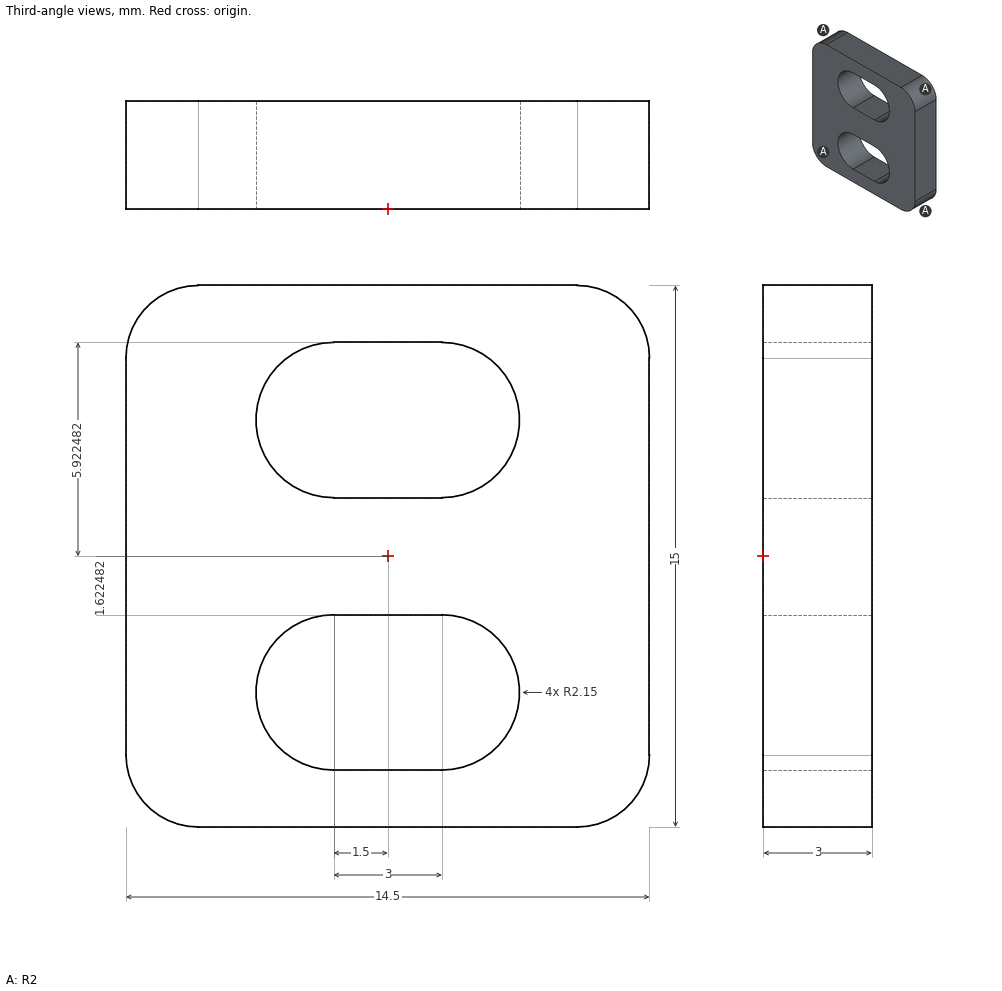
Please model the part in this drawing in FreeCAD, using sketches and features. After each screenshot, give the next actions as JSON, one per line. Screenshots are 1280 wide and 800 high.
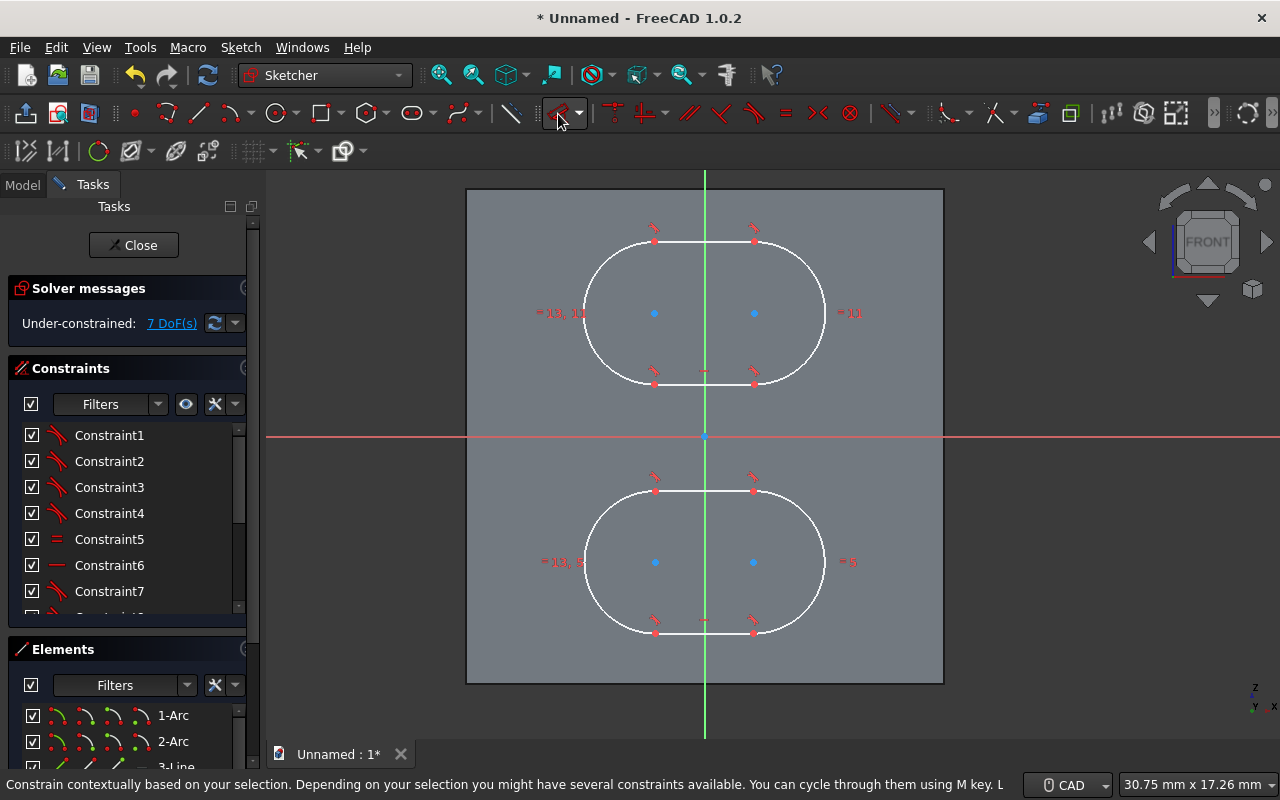
{"action": "left_click", "coordinate": [598, 520]}
{"action": "left_click", "coordinate": [572, 501]}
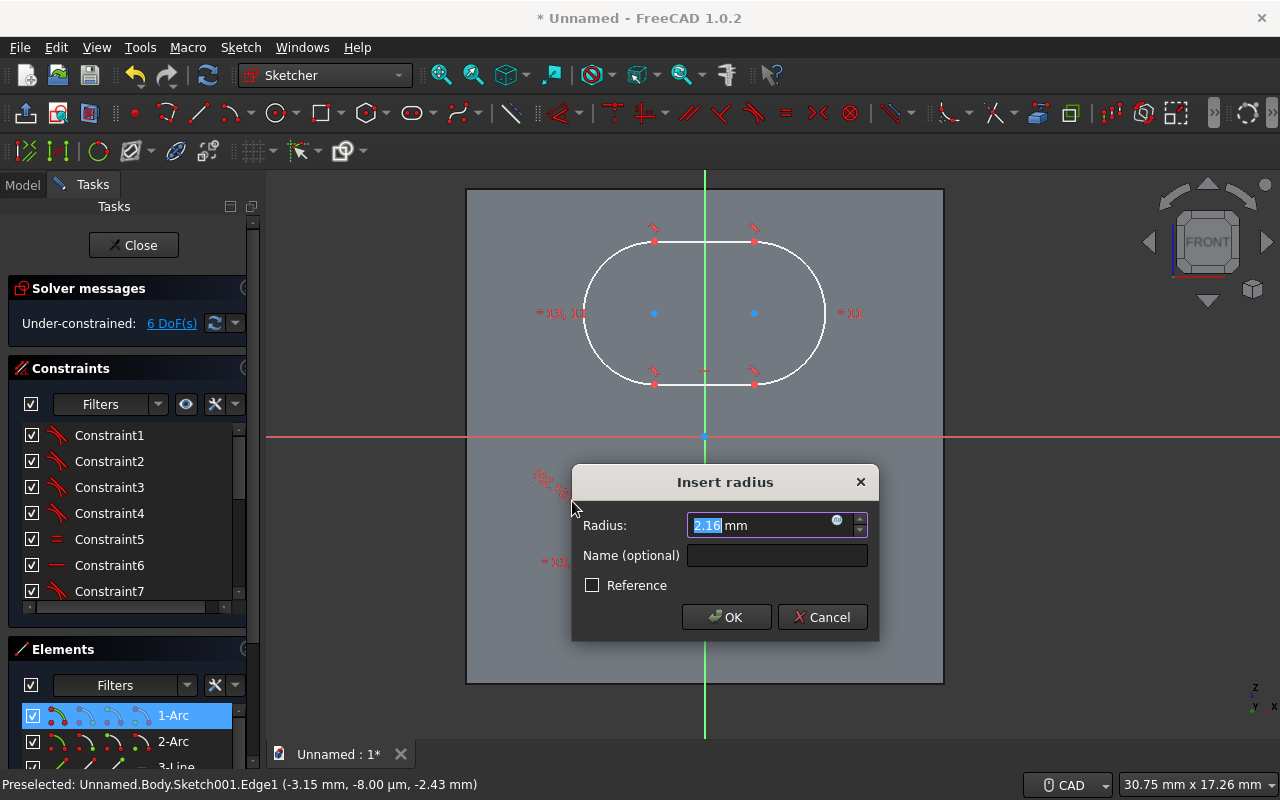
{"action": "type", "text": "2.15"}
{"action": "key", "text": "Return"}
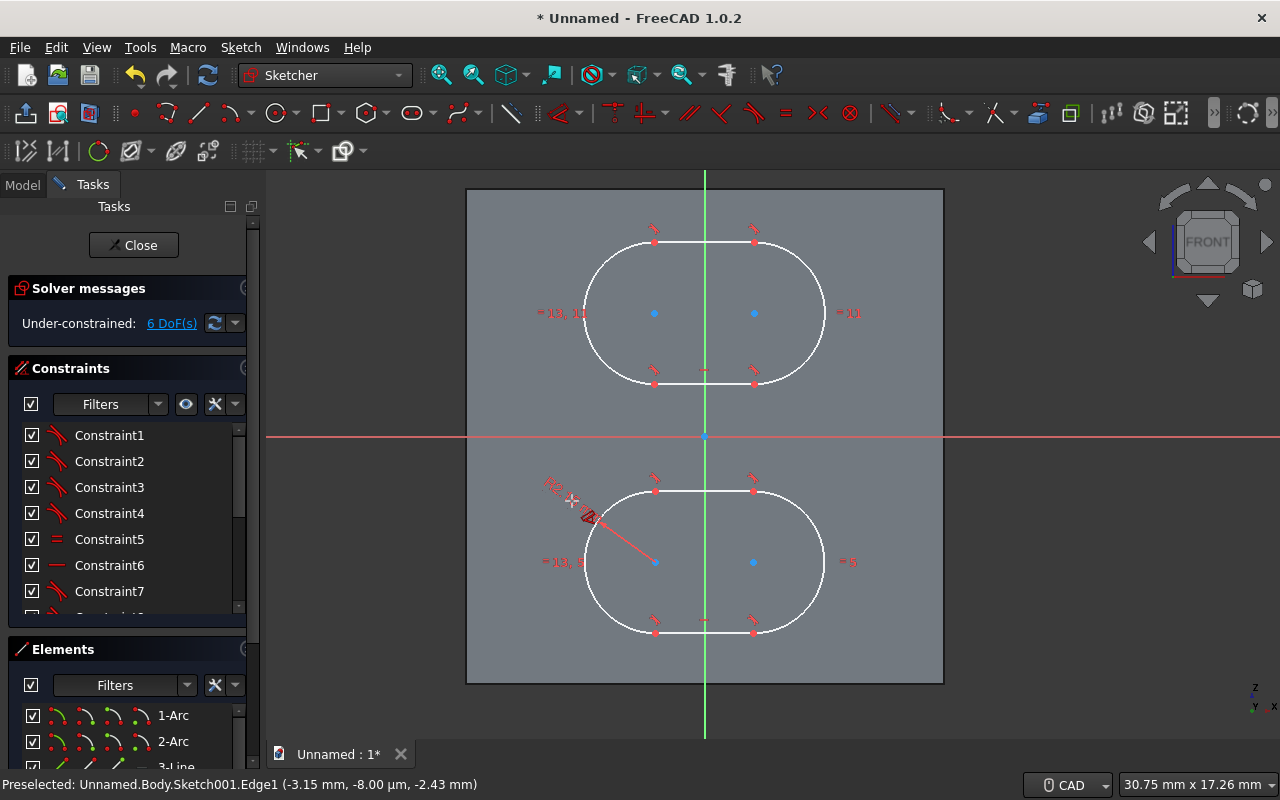
{"action": "left_click", "coordinate": [685, 491]}
{"action": "left_click", "coordinate": [682, 525]}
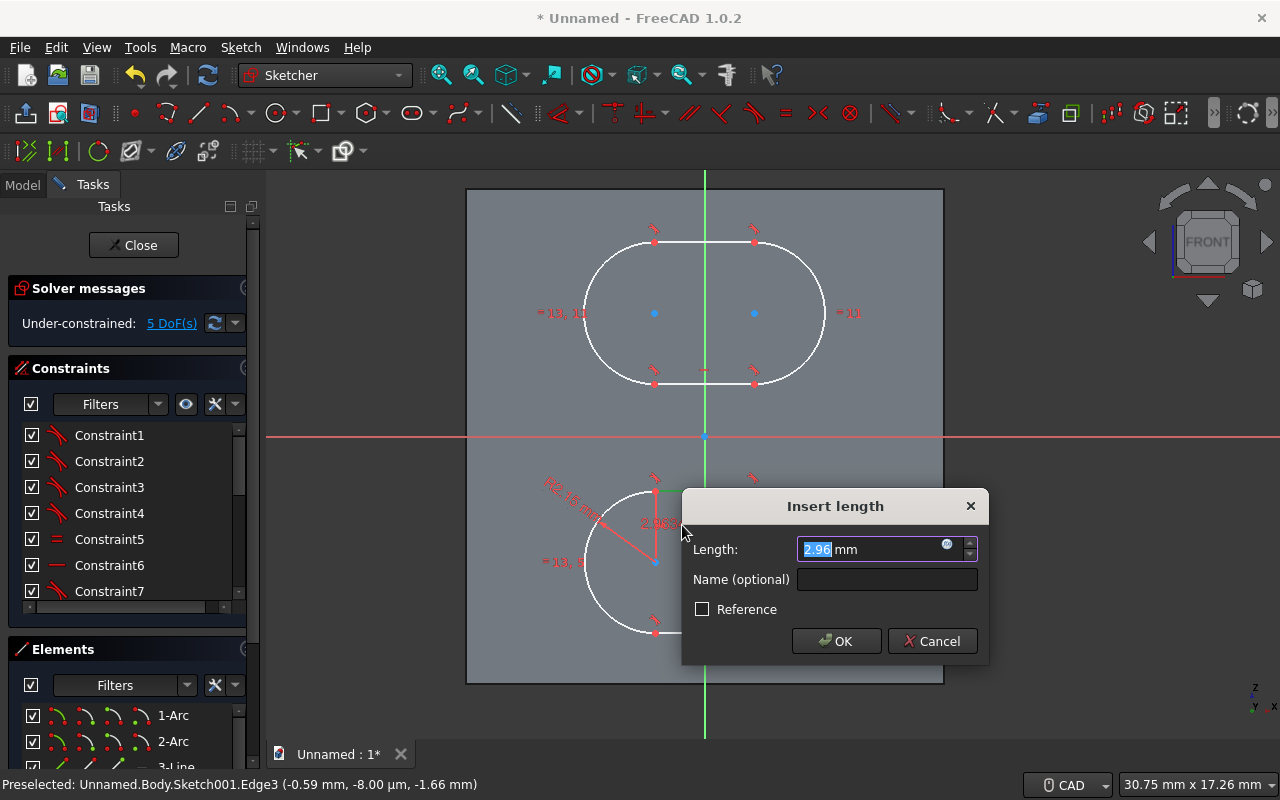
{"action": "type", "text": "3"}
{"action": "key", "text": "Return"}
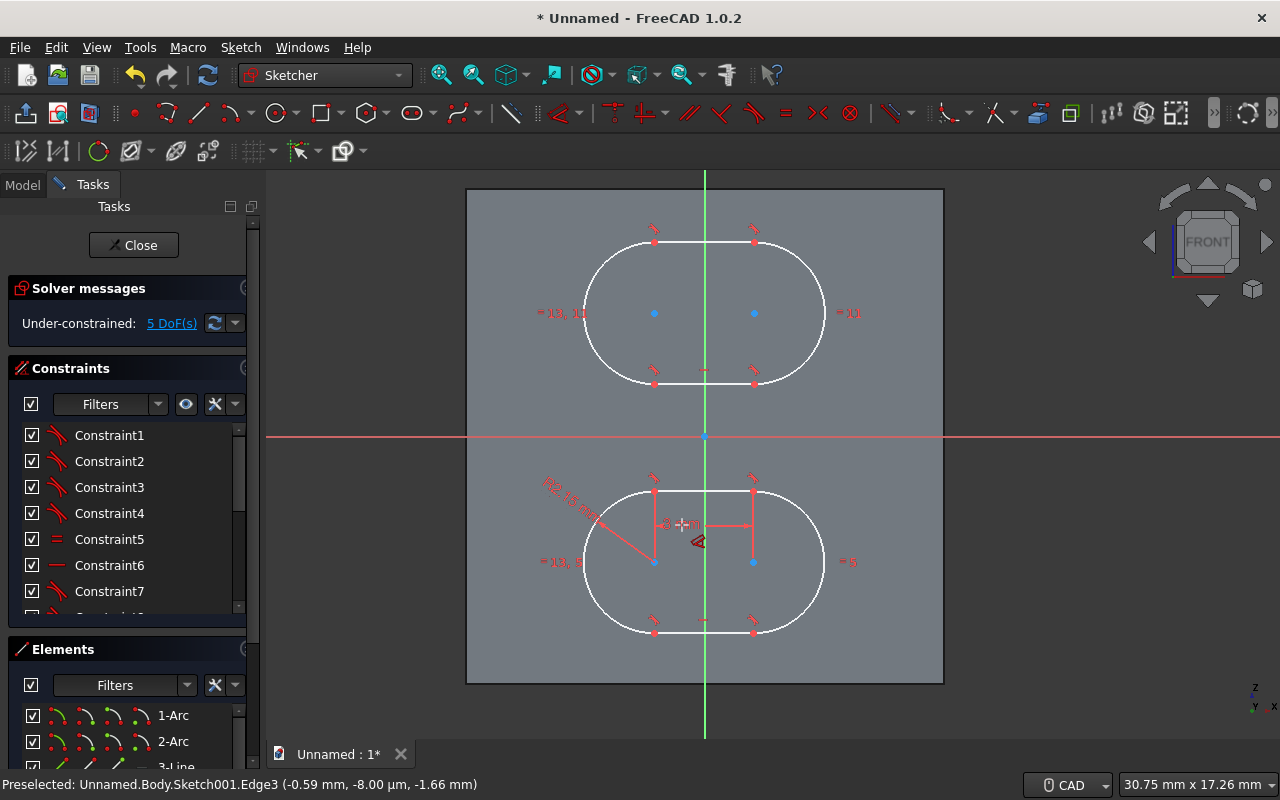
{"action": "left_click", "coordinate": [685, 242]}
{"action": "left_click", "coordinate": [682, 208]}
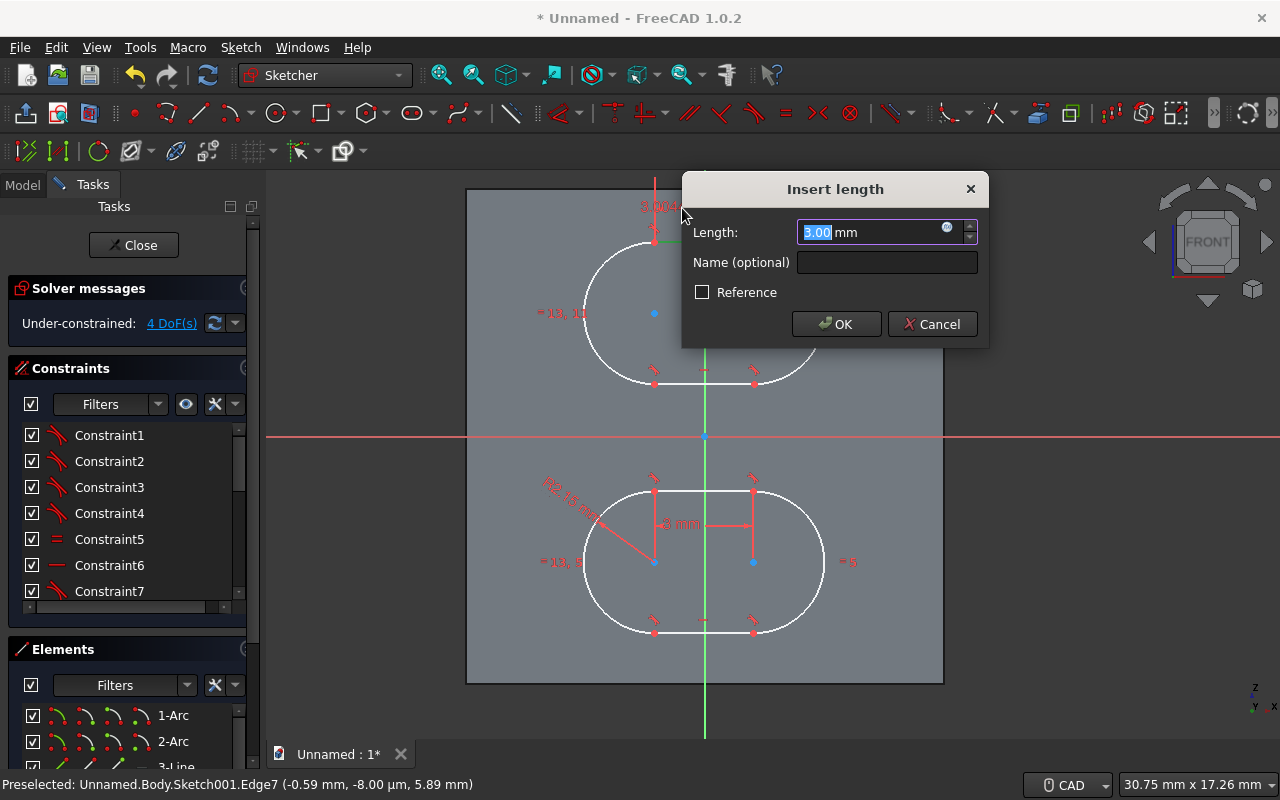
{"action": "type", "text": "3"}
{"action": "key", "text": "Return"}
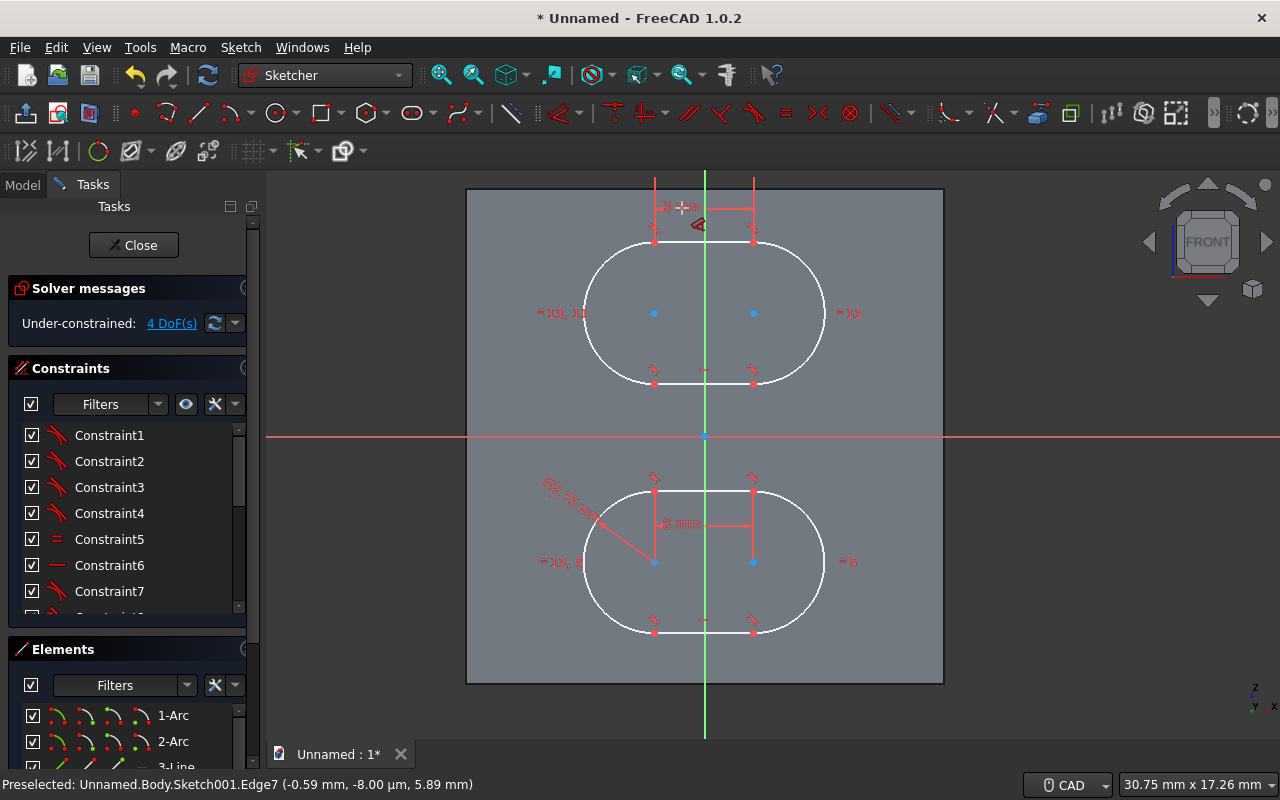
{"action": "left_click", "coordinate": [655, 491]}
{"action": "left_click", "coordinate": [680, 403]}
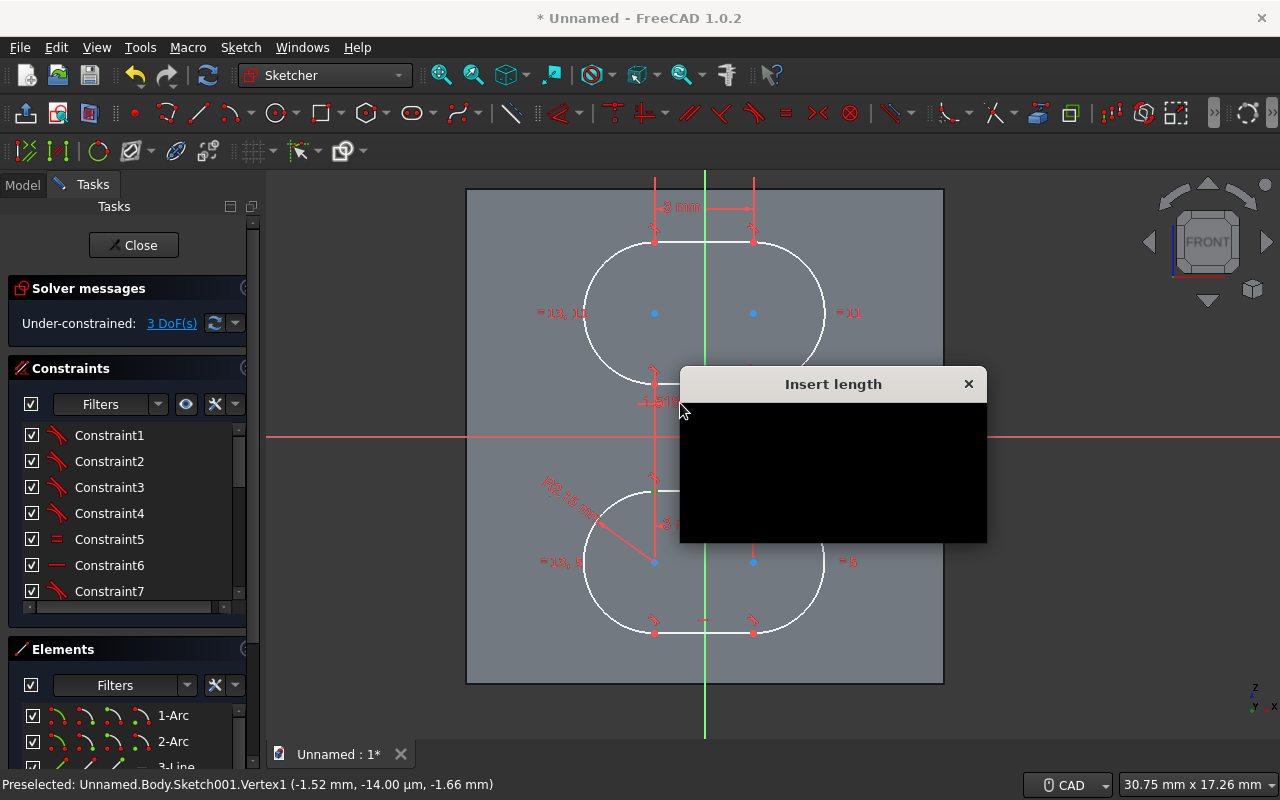
{"action": "type", "text": "1.5"}
{"action": "key", "text": "Return"}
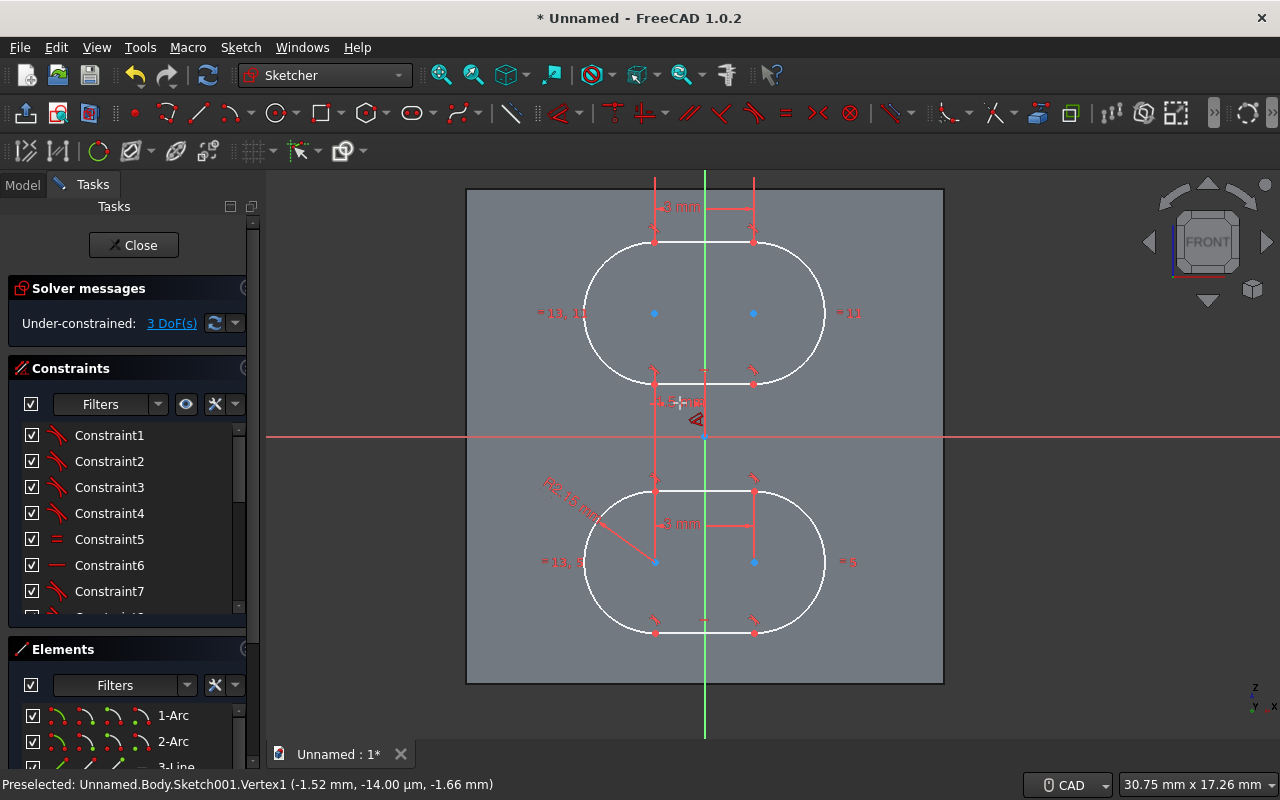
{"action": "left_click", "coordinate": [655, 242]}
{"action": "left_click", "coordinate": [680, 471]}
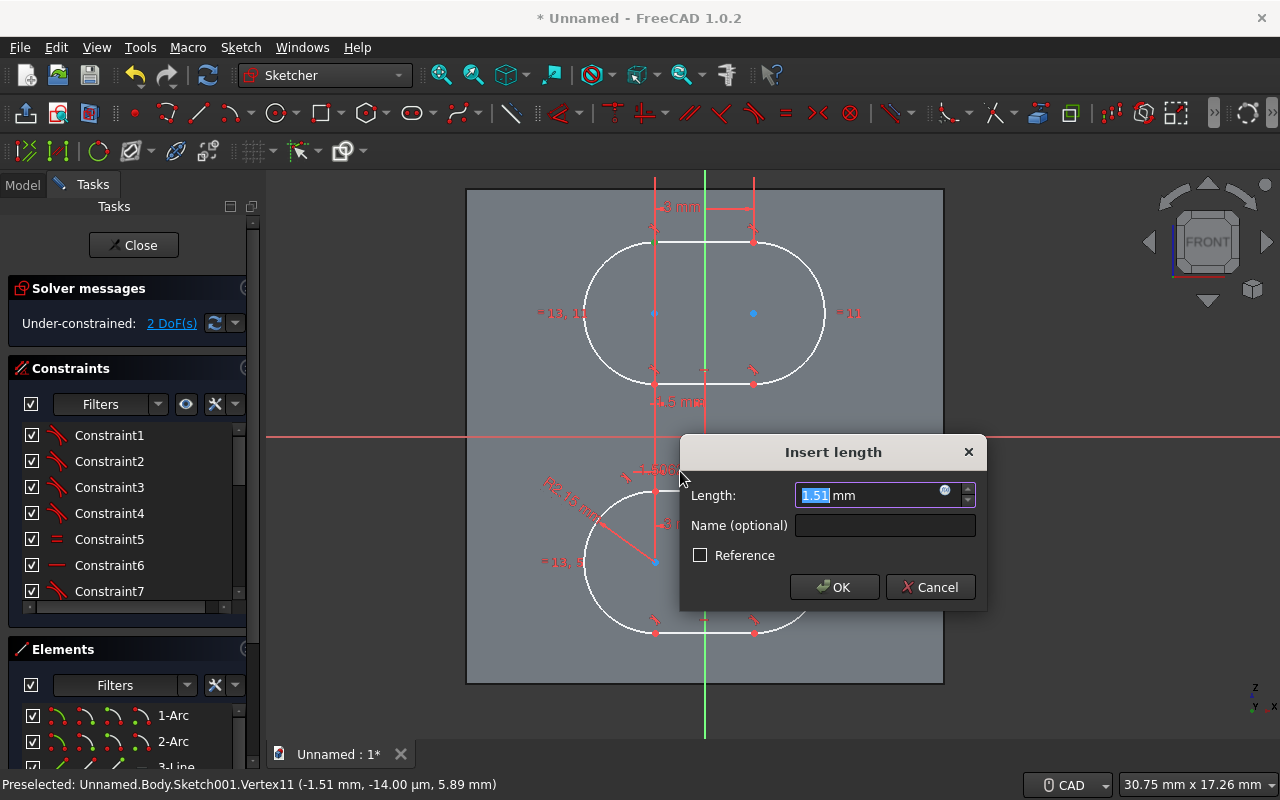
{"action": "type", "text": "1.5"}
{"action": "key", "text": "Return"}